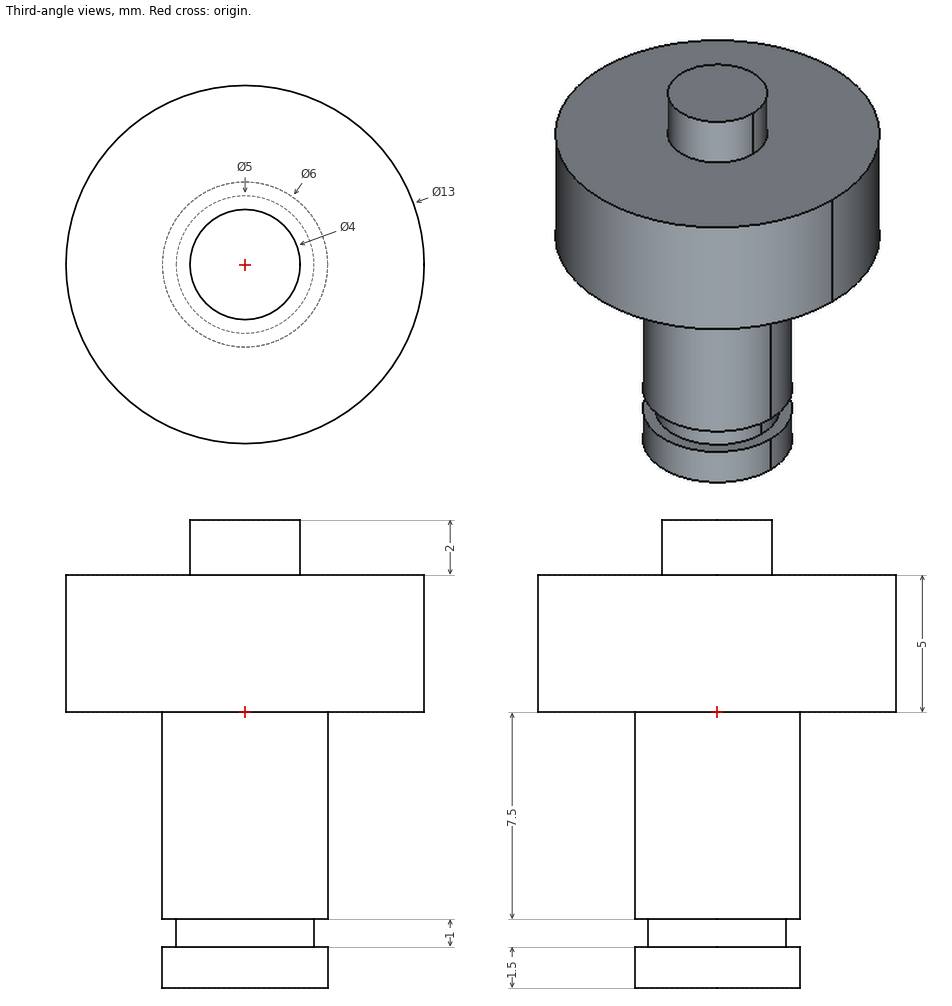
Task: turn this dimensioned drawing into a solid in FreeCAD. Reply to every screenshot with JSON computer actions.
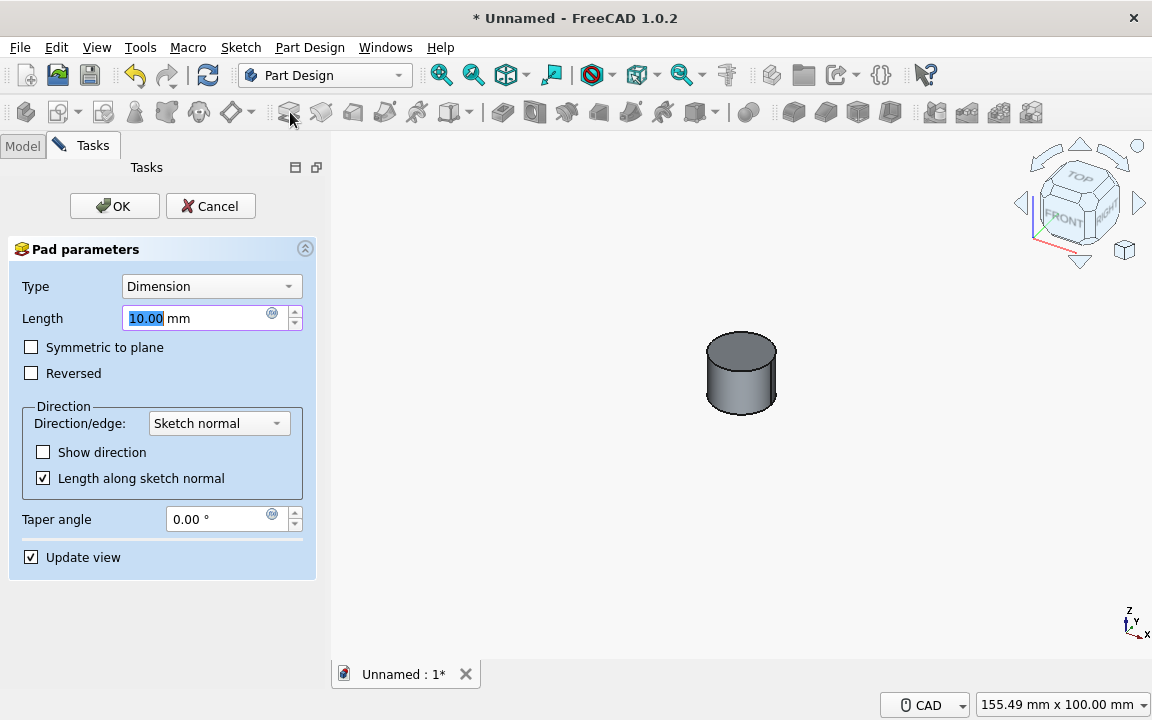
{"action": "type", "text": "5"}
{"action": "key", "text": "Tab"}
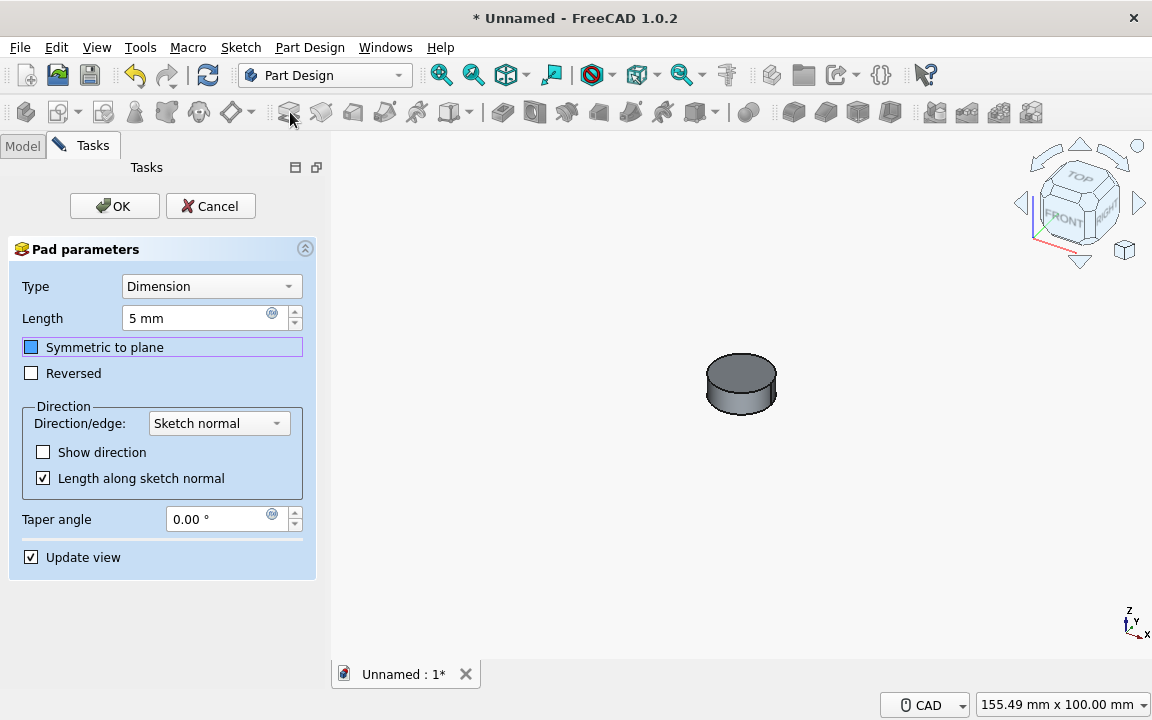
{"action": "left_click", "coordinate": [115, 206]}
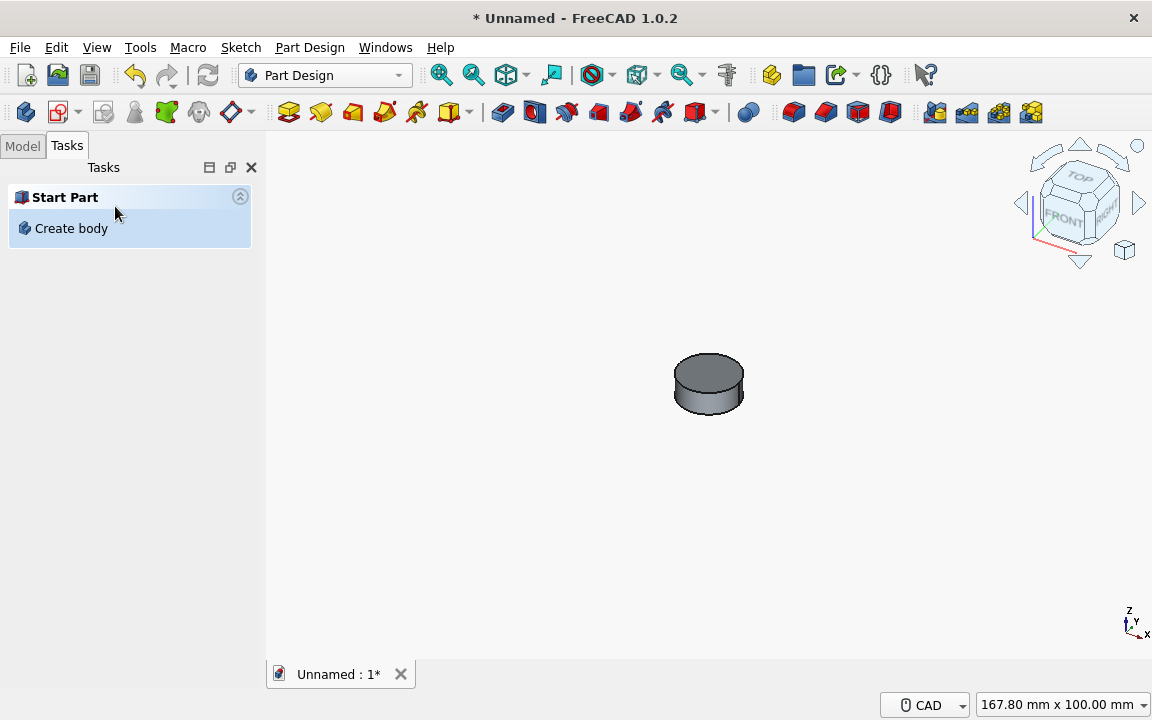
{"action": "key", "text": "v f"}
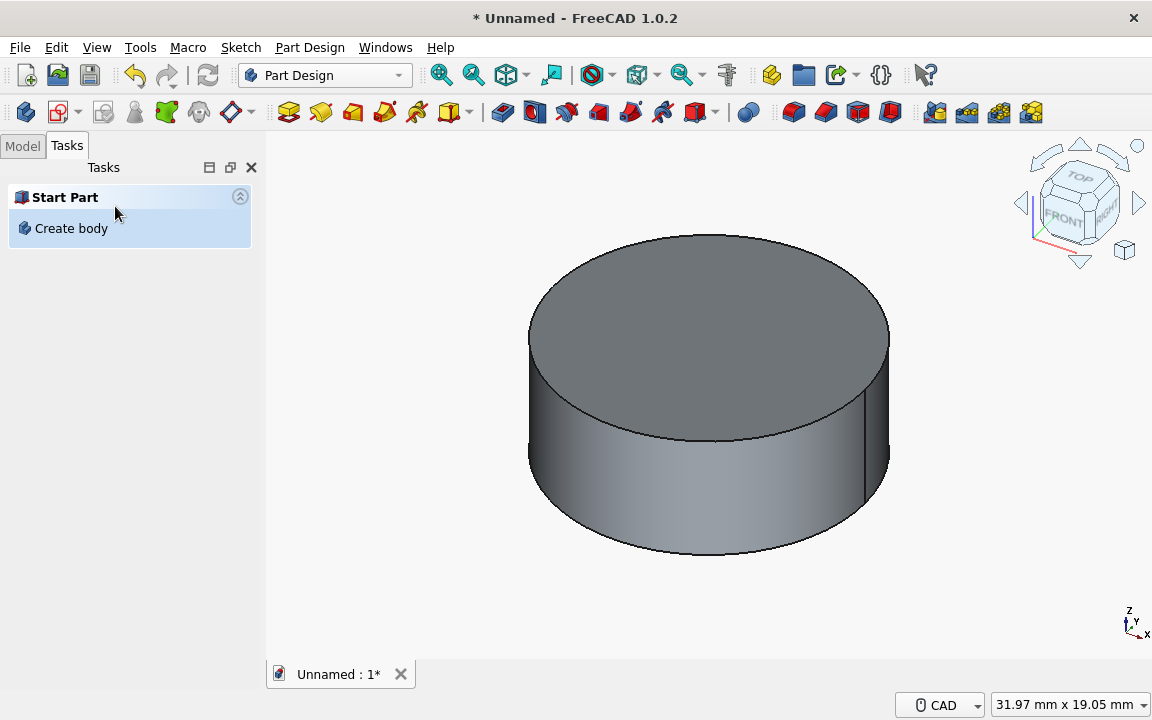
{"action": "left_click", "coordinate": [709, 337]}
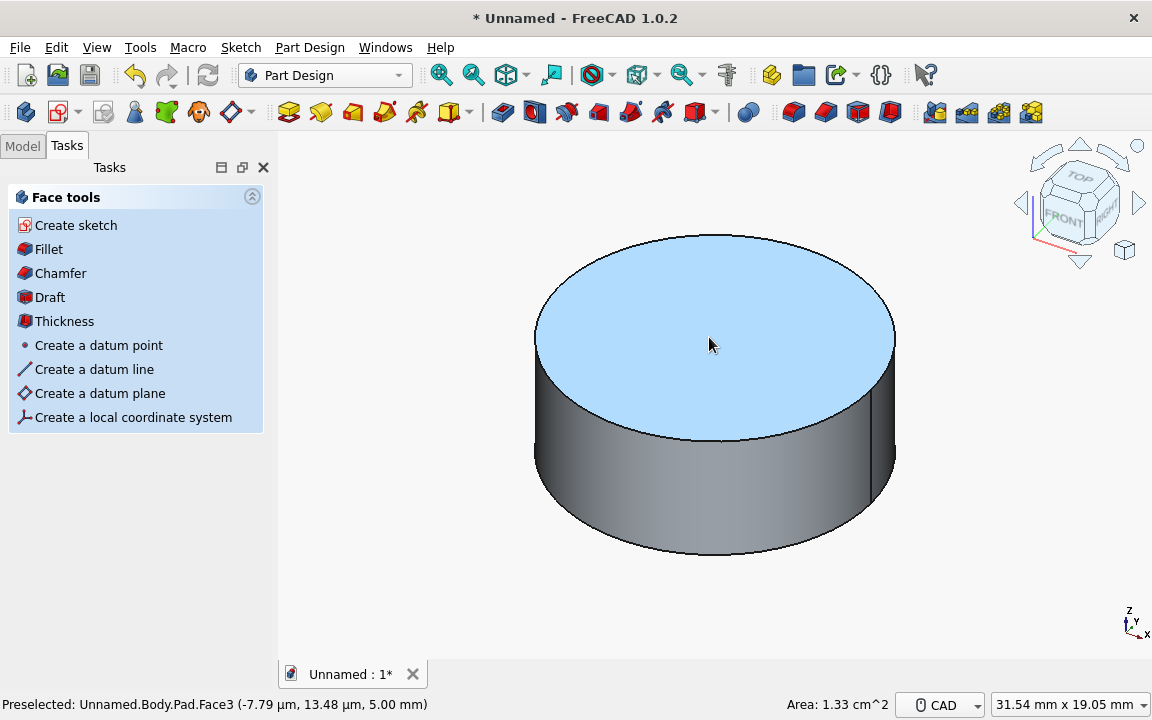
{"action": "left_click", "coordinate": [58, 112]}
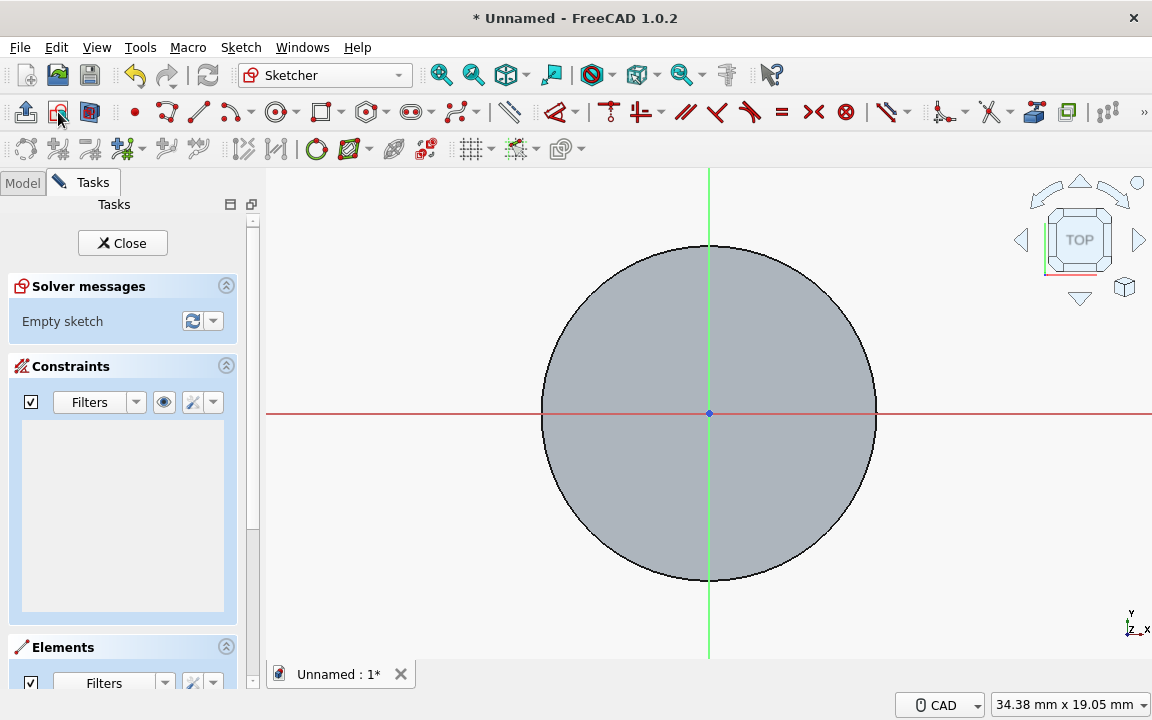
{"action": "scroll", "coordinate": [749, 414], "scroll_direction": "up", "scroll_amount": 5}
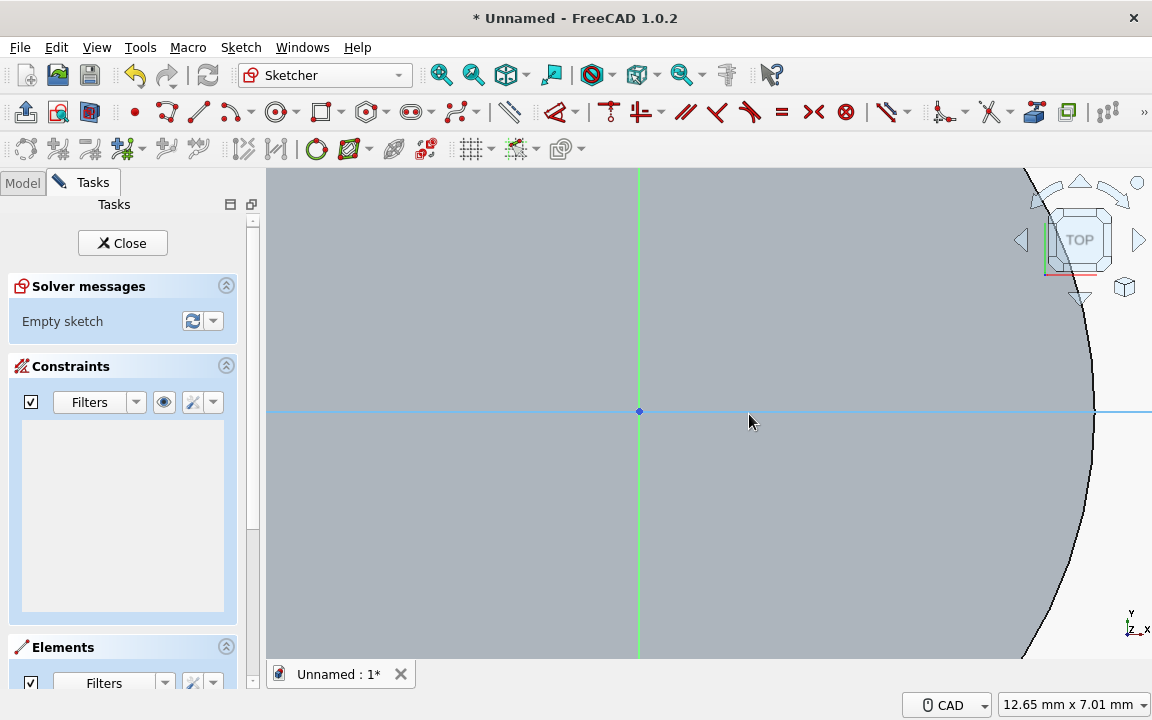
{"action": "key", "text": "g c"}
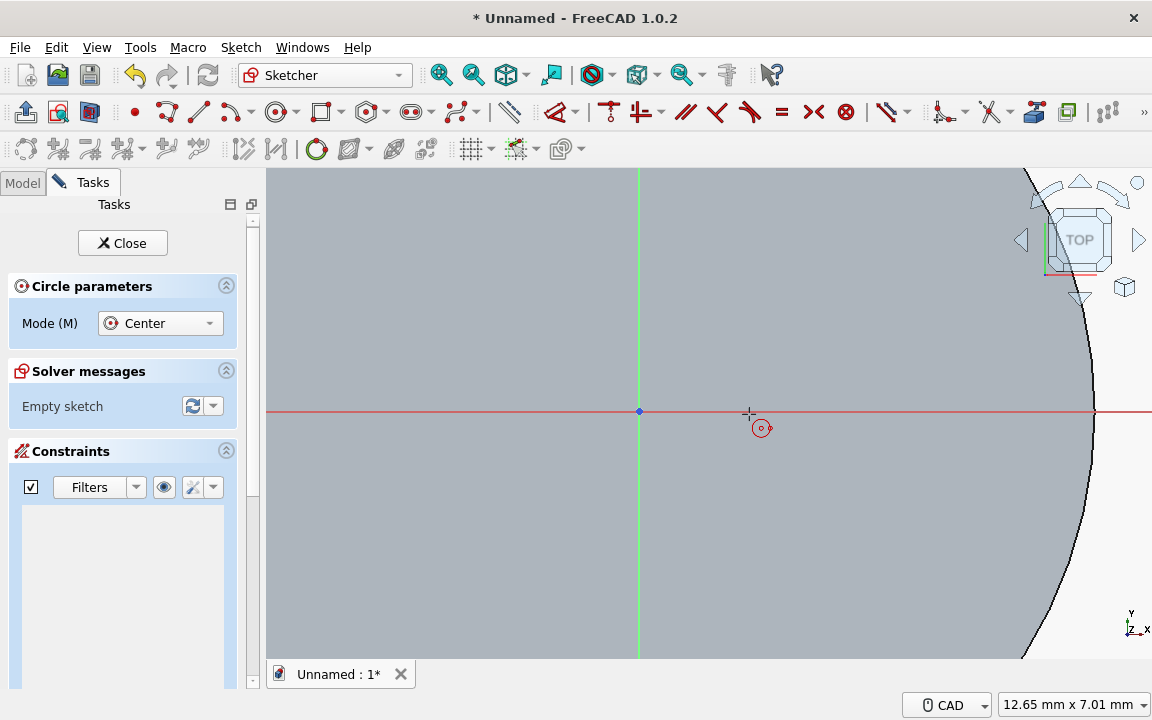
{"action": "left_click", "coordinate": [639, 412]}
{"action": "left_click", "coordinate": [738, 313]}
{"action": "key", "text": "Escape"}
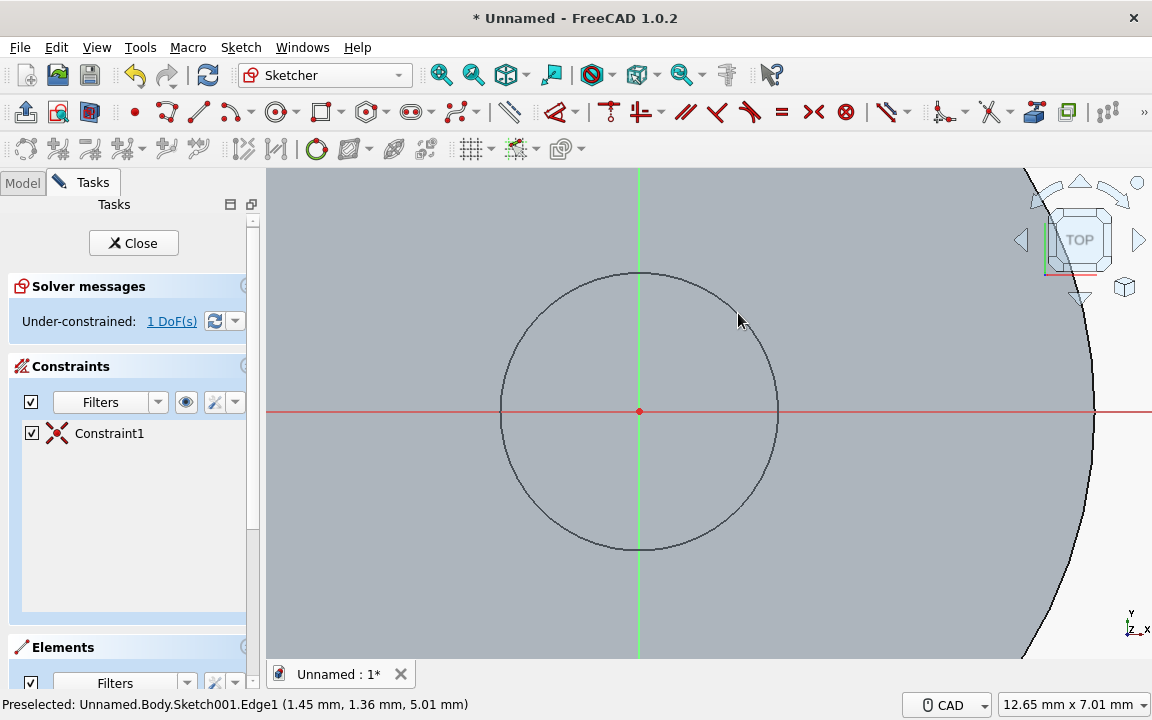
{"action": "key", "text": "d"}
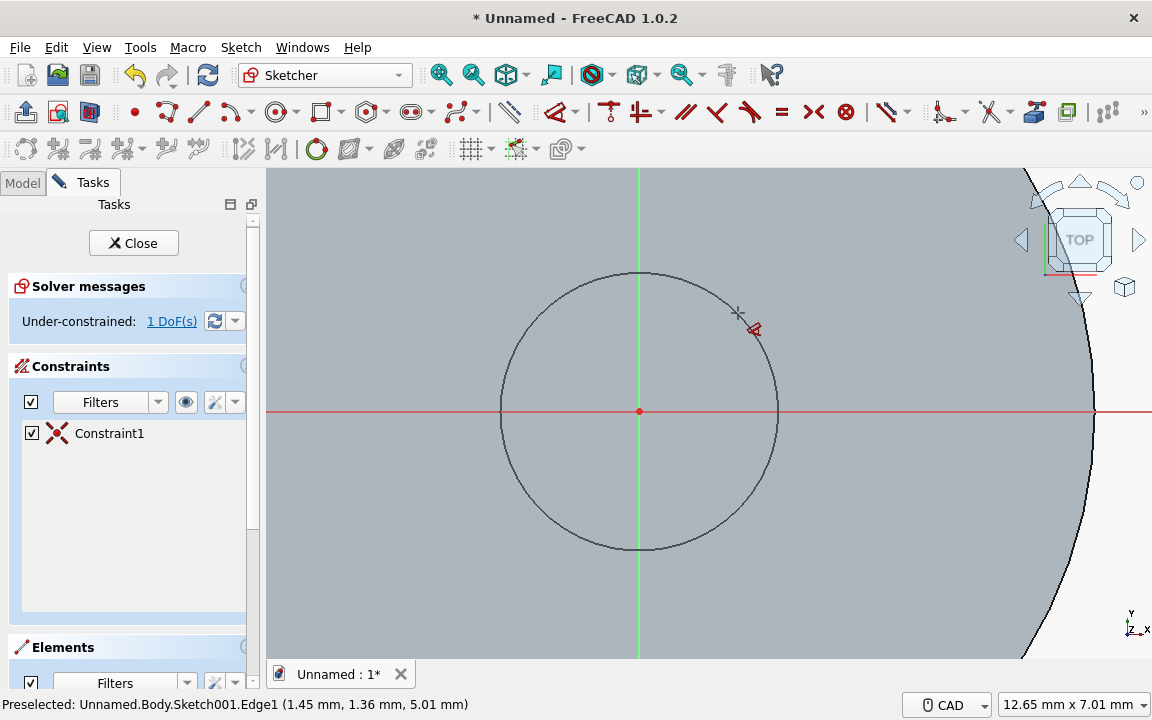
{"action": "left_click", "coordinate": [737, 313]}
{"action": "left_click", "coordinate": [759, 290]}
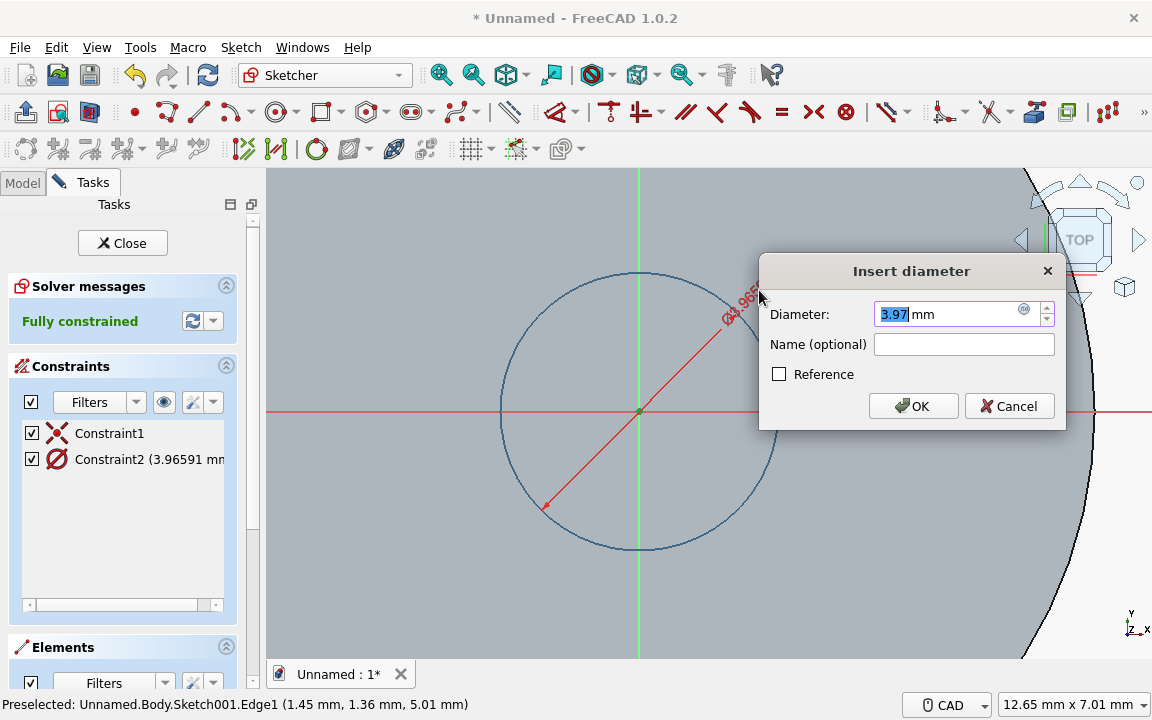
{"action": "type", "text": "4"}
{"action": "key", "text": "Return"}
{"action": "key", "text": "Escape"}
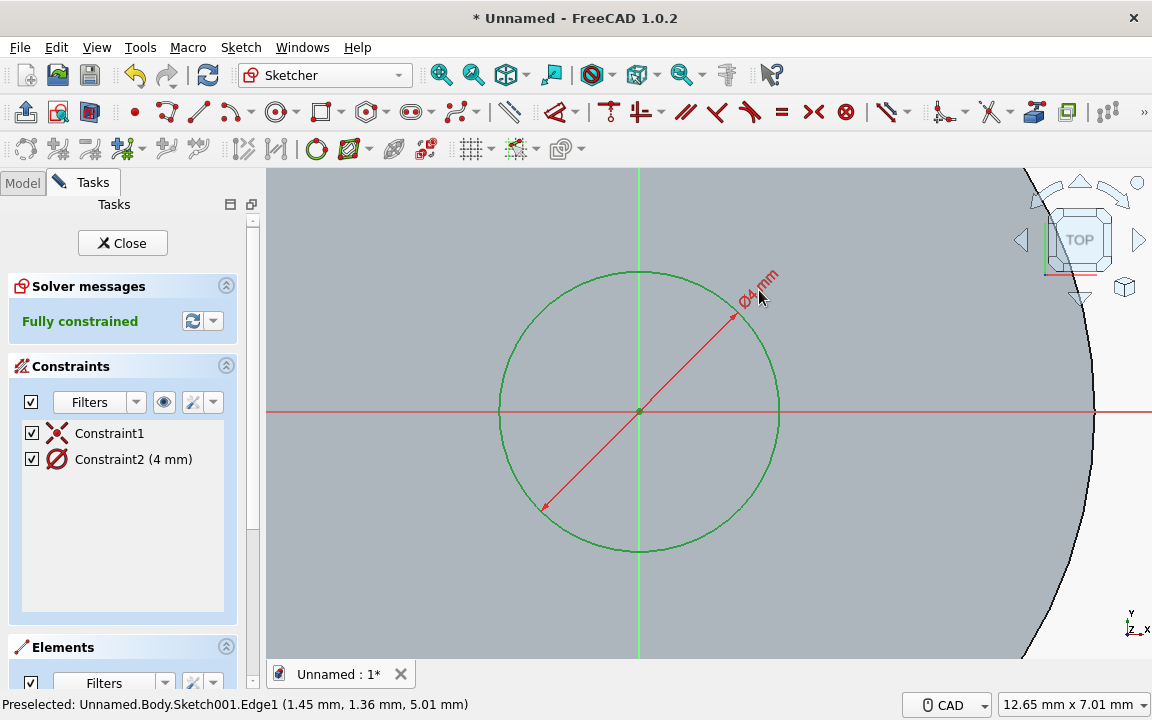
{"action": "left_click", "coordinate": [123, 243]}